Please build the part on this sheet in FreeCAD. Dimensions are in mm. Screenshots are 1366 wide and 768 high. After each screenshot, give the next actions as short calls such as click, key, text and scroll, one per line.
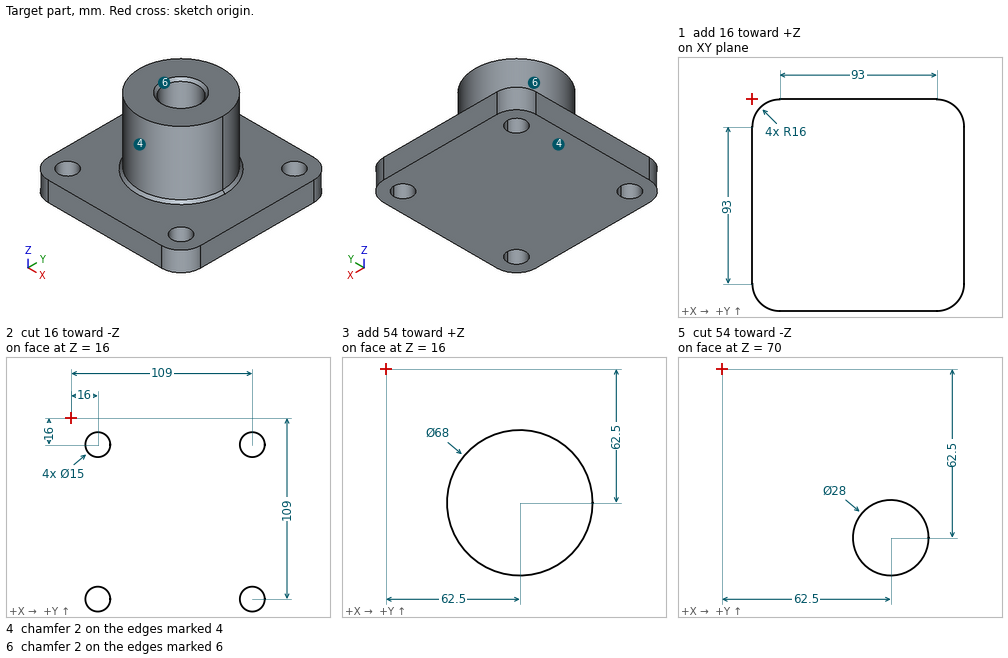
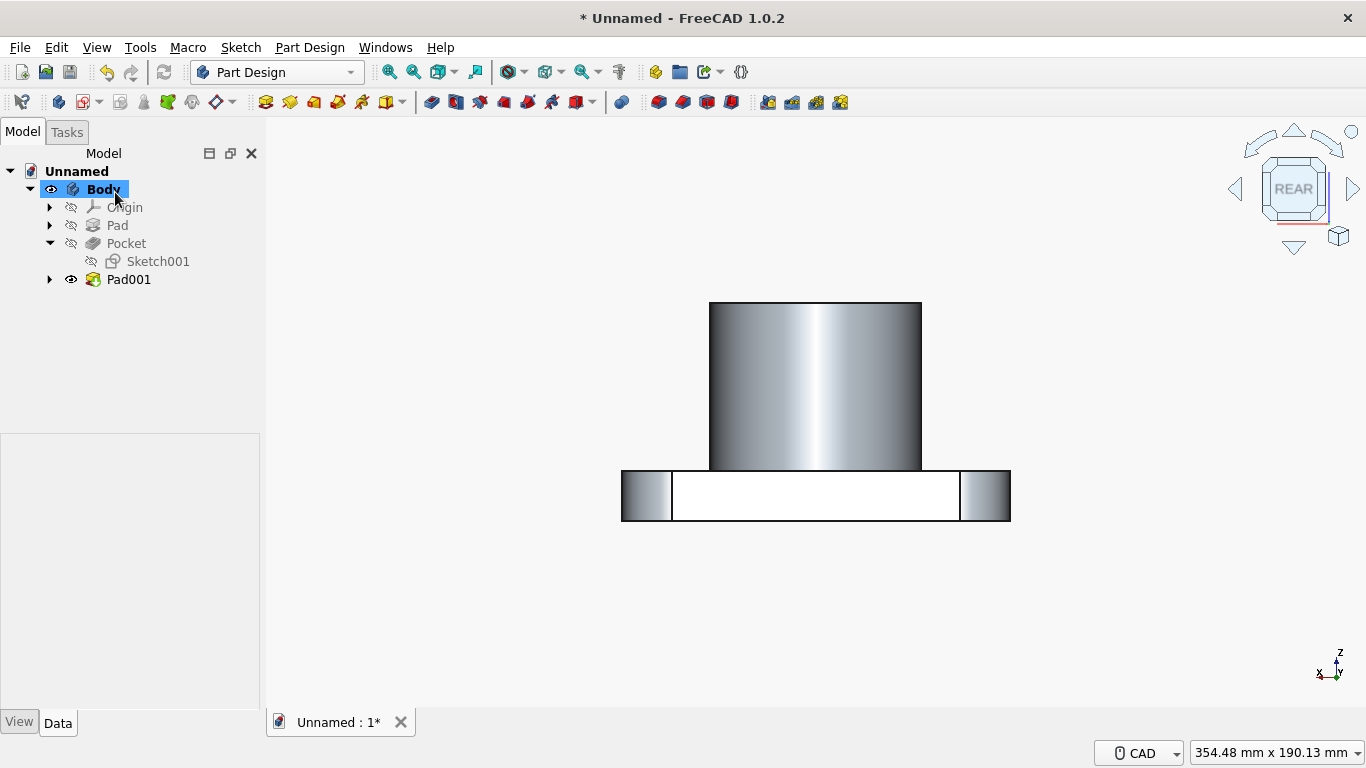
key(6)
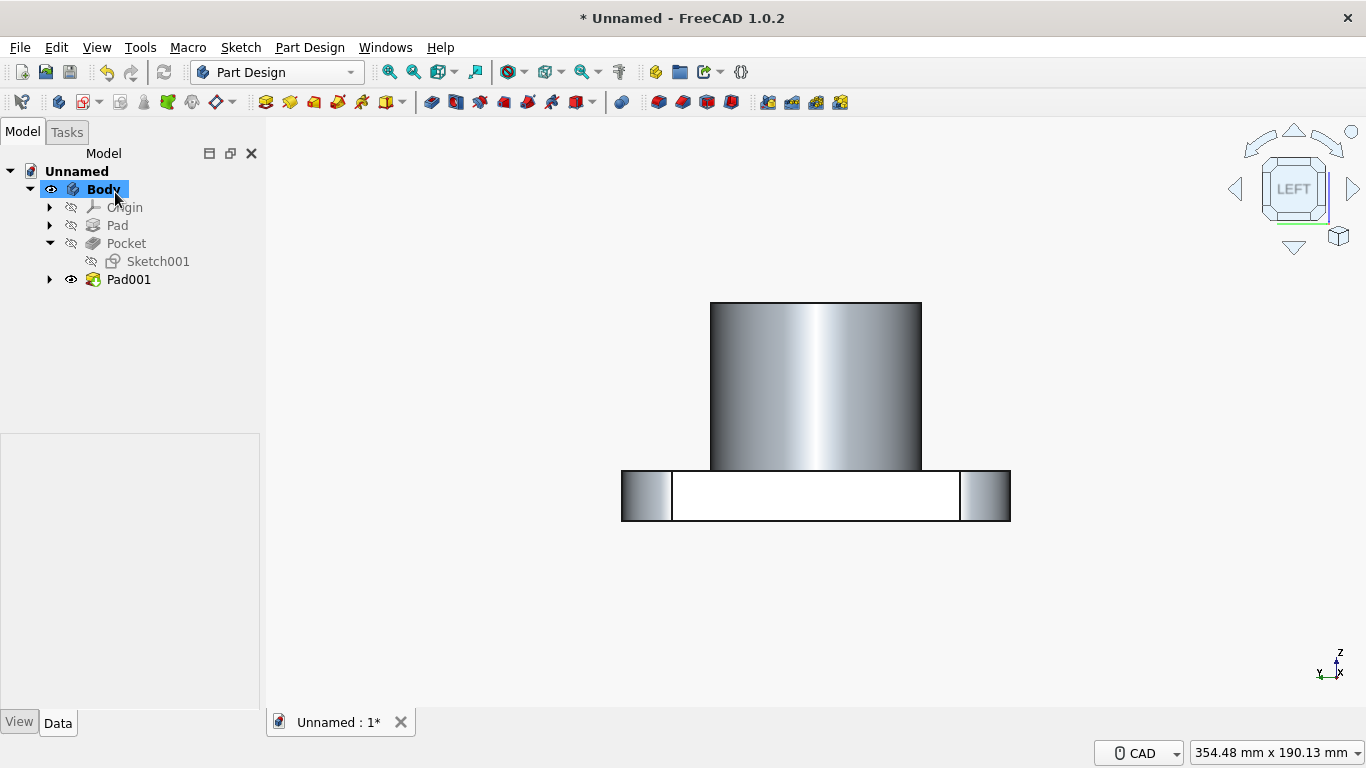
click(390, 72)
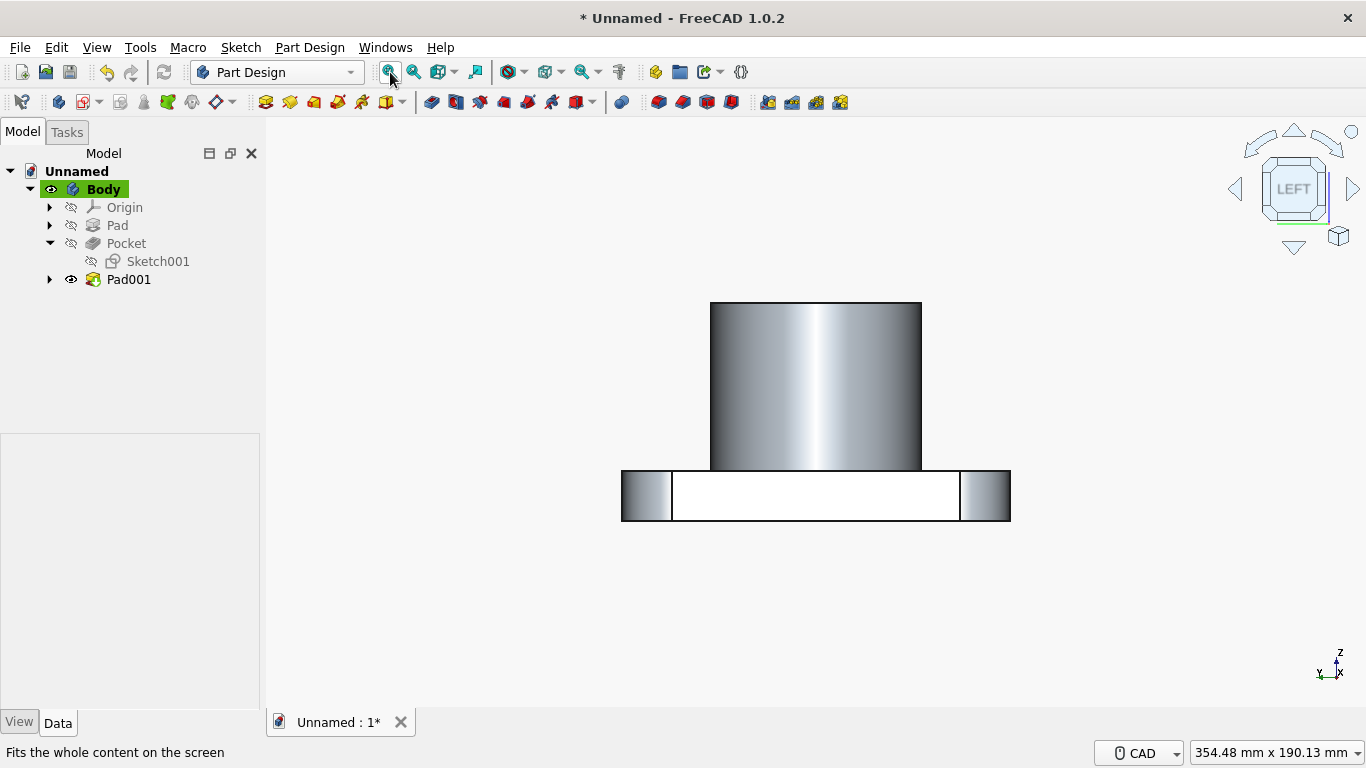
key(v)
key(3)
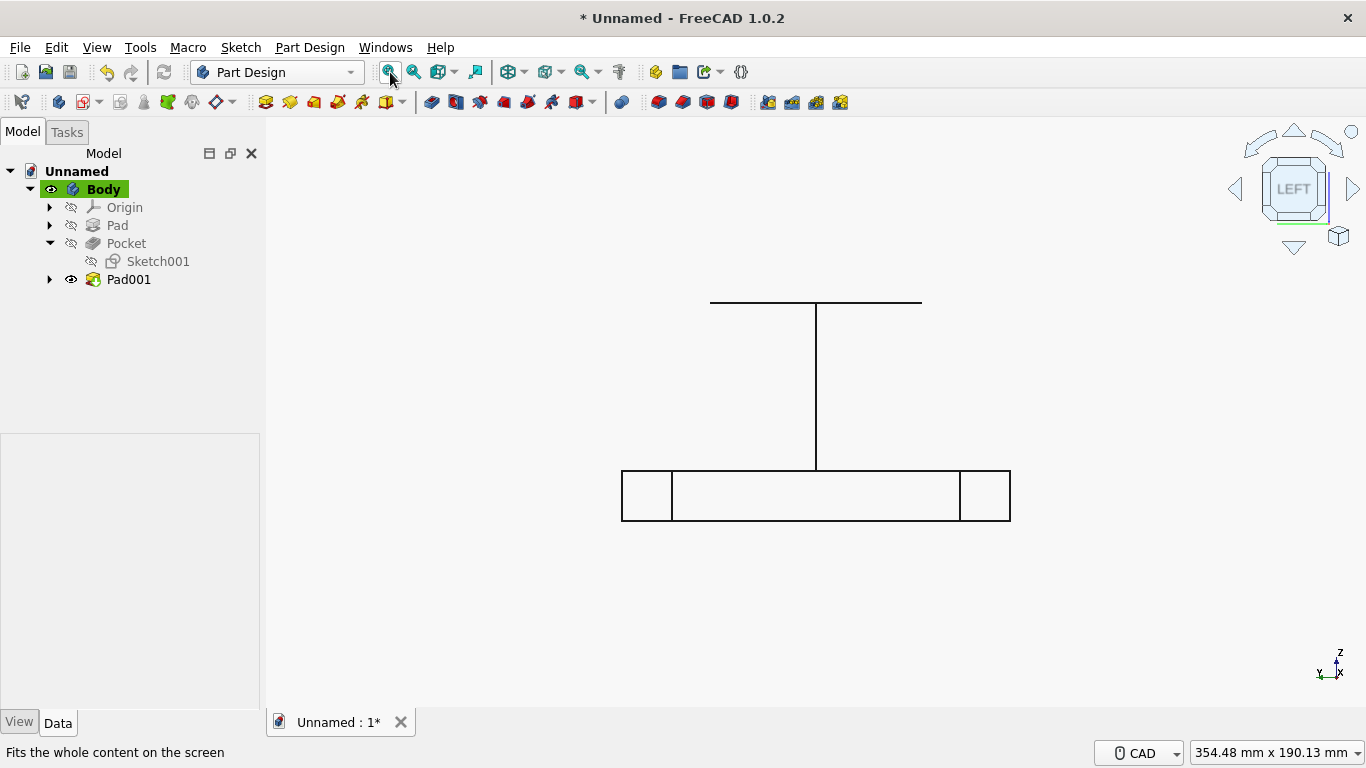
key(0)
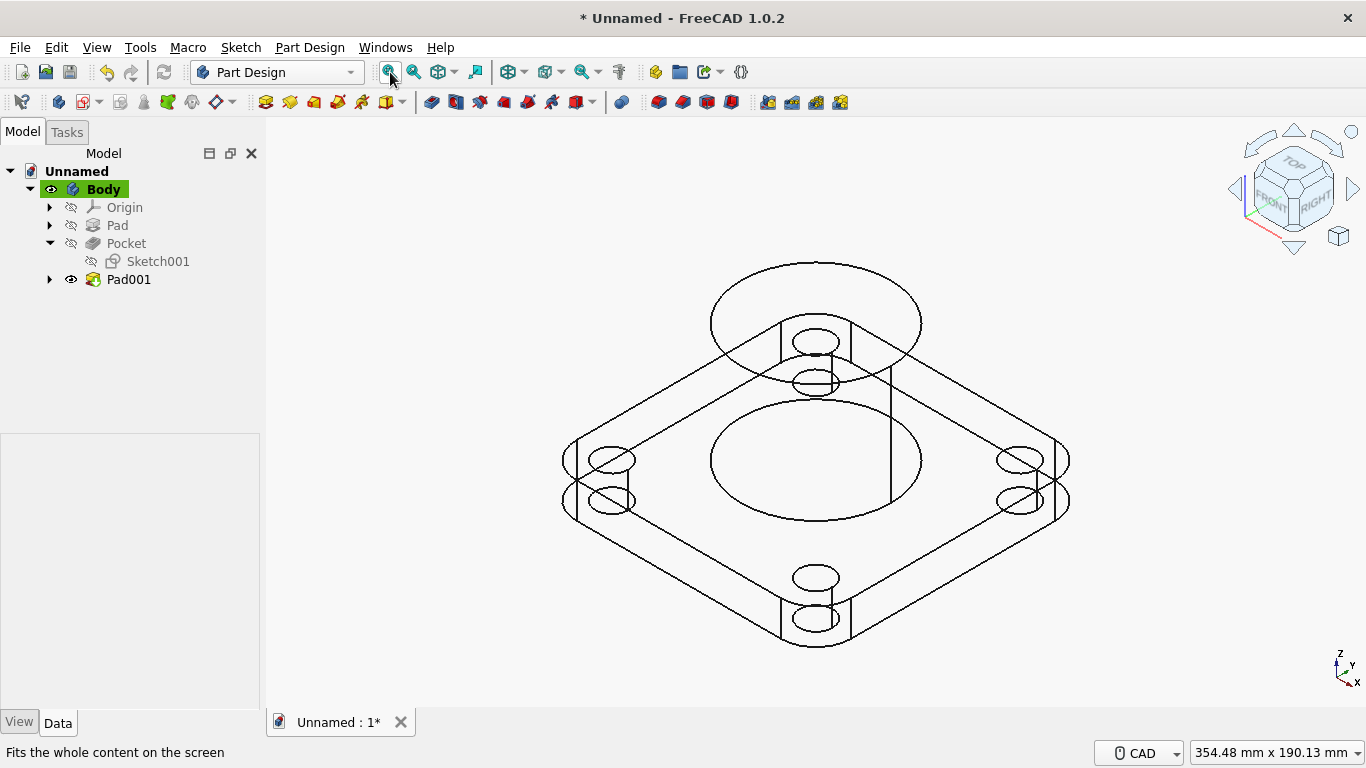
click(741, 416)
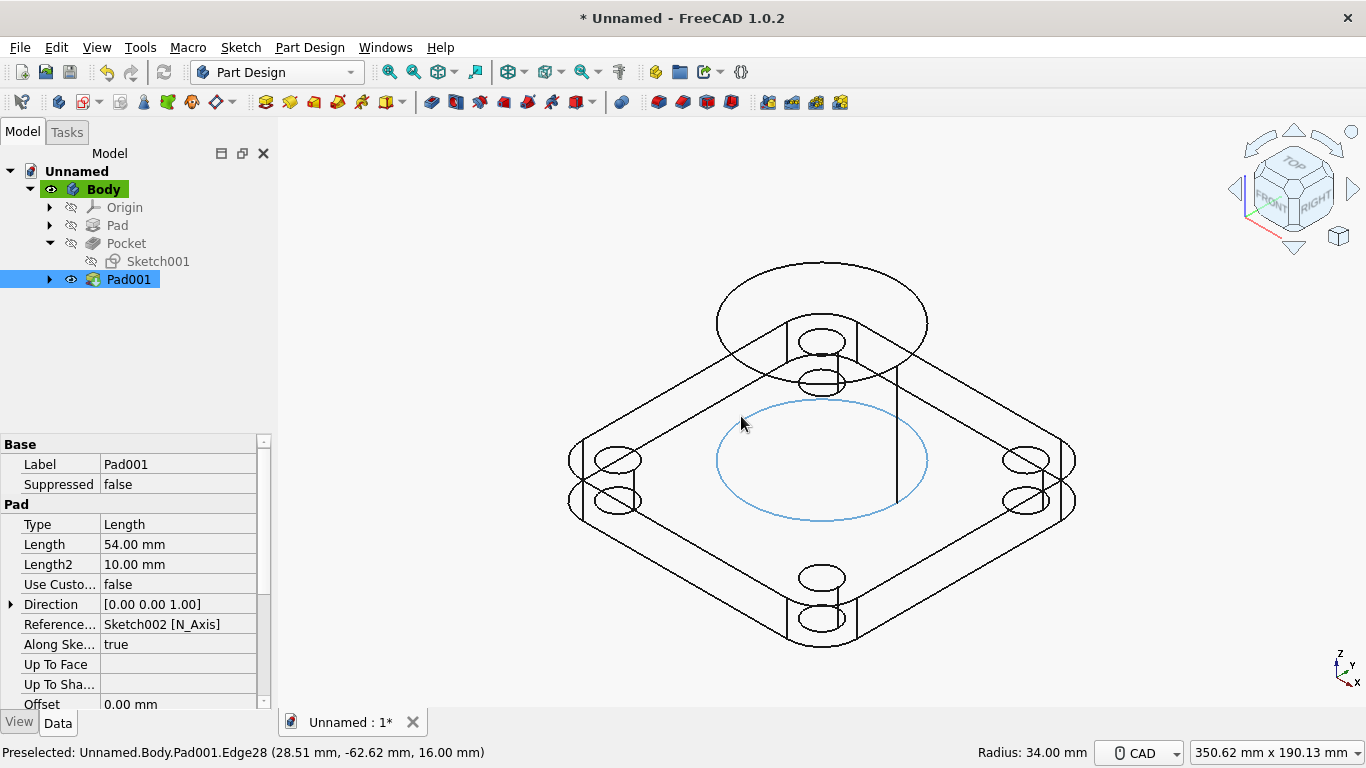
key(v)
key(1)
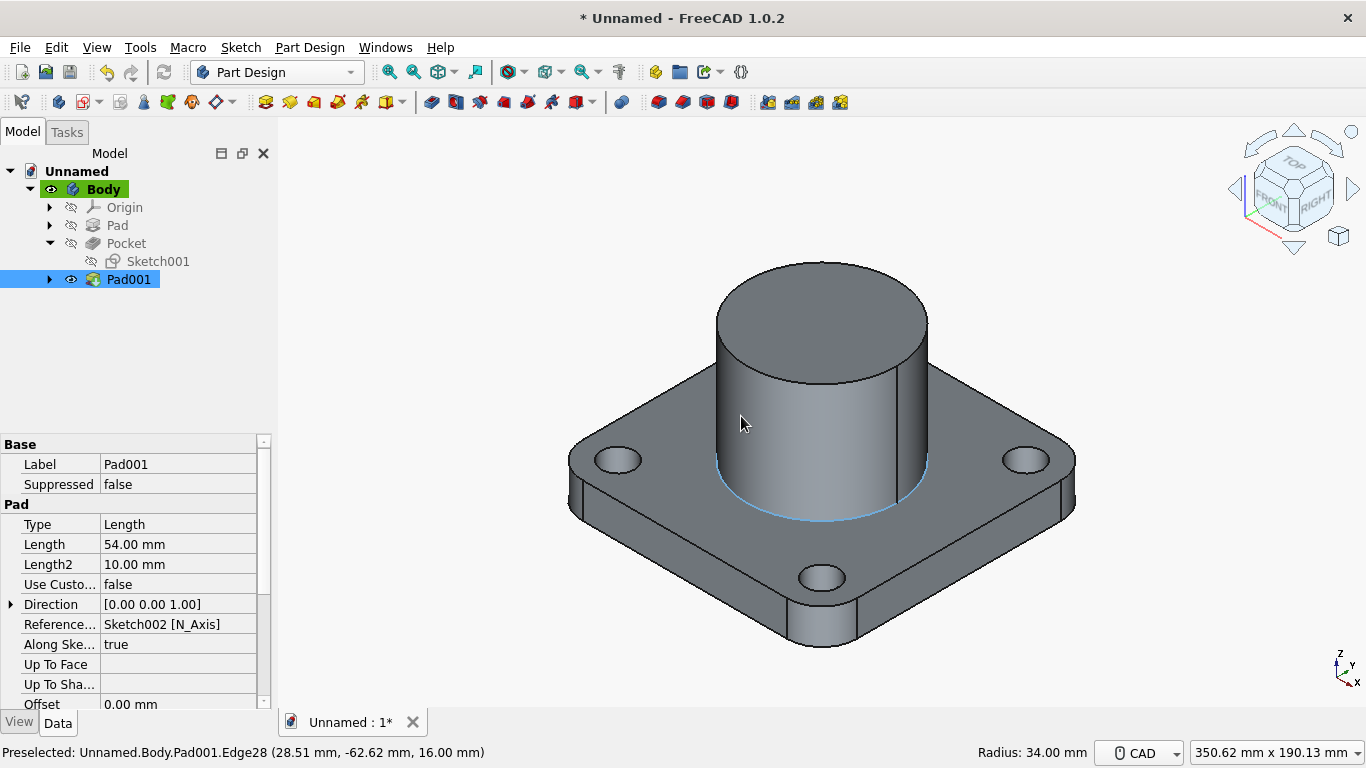
click(684, 102)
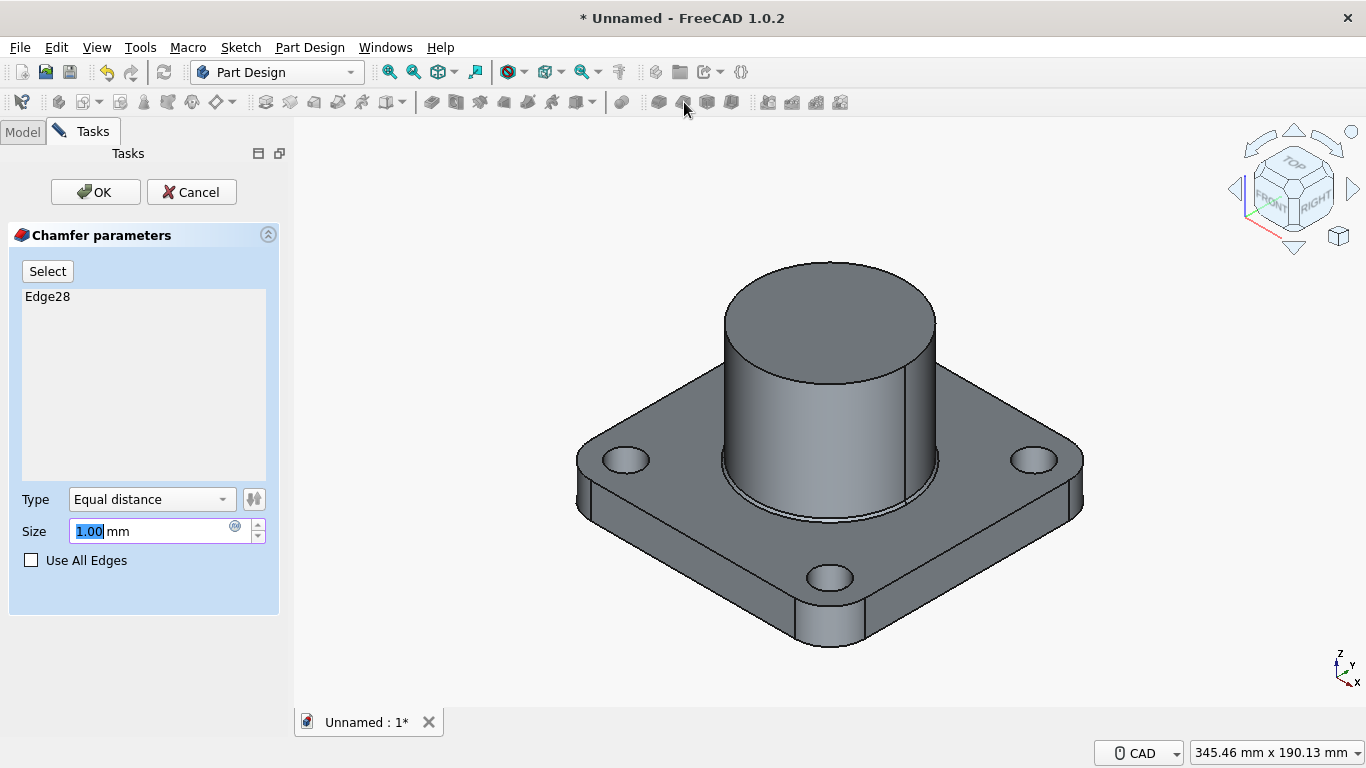
text(2)
key(Tab)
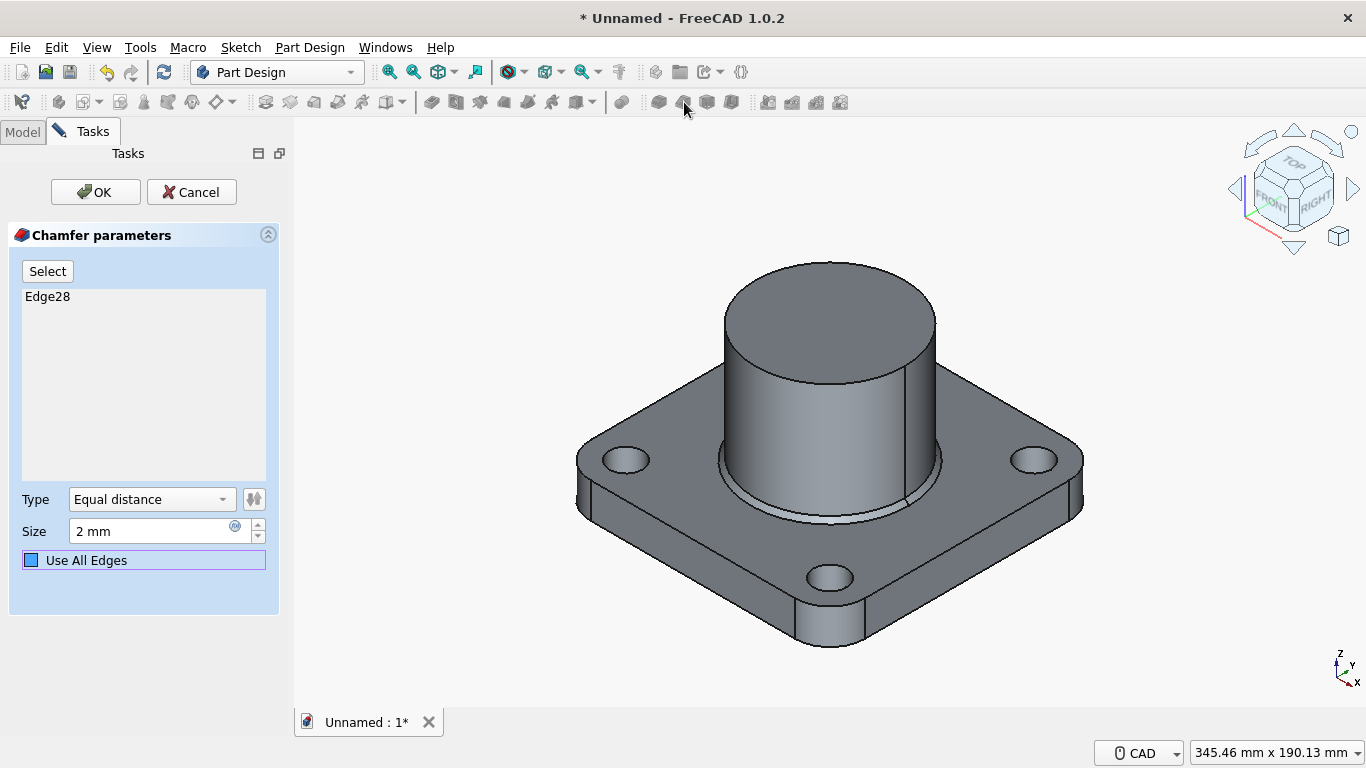
click(96, 192)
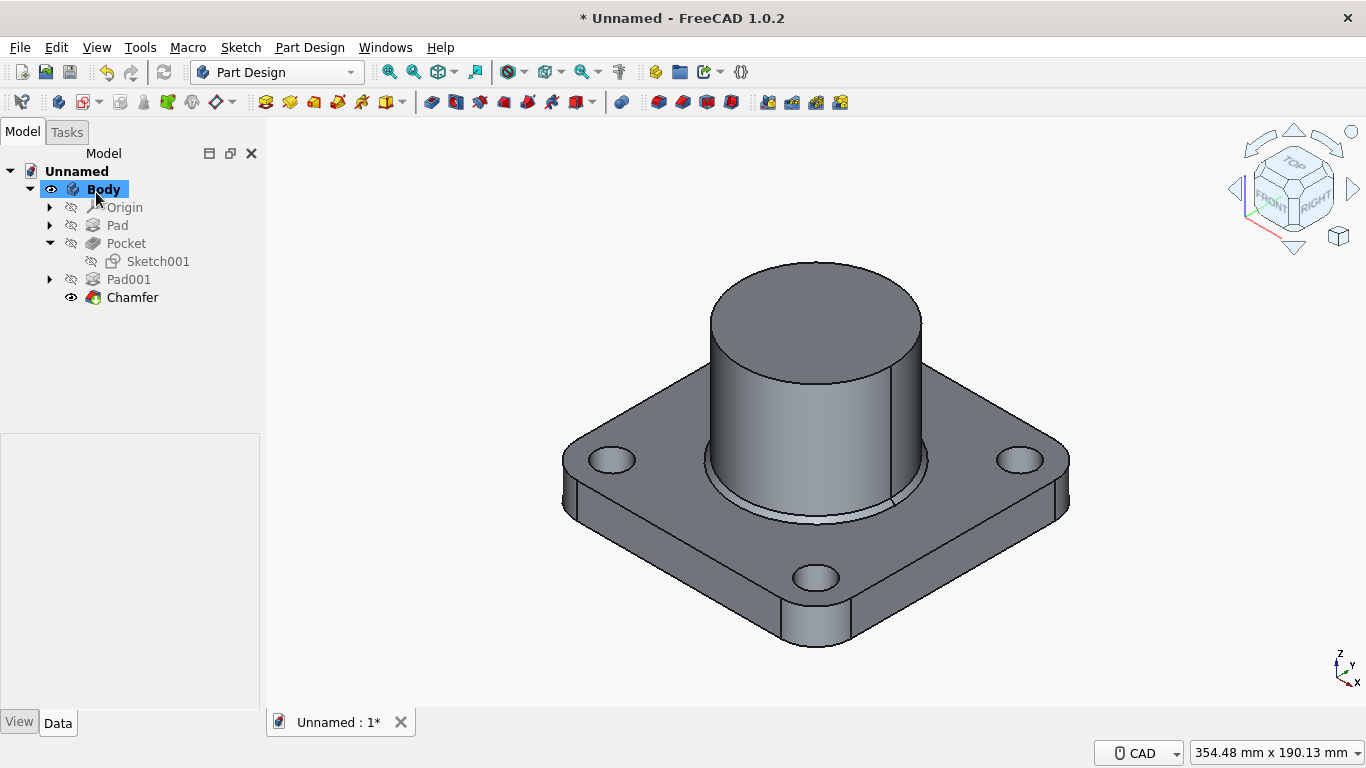
click(816, 322)